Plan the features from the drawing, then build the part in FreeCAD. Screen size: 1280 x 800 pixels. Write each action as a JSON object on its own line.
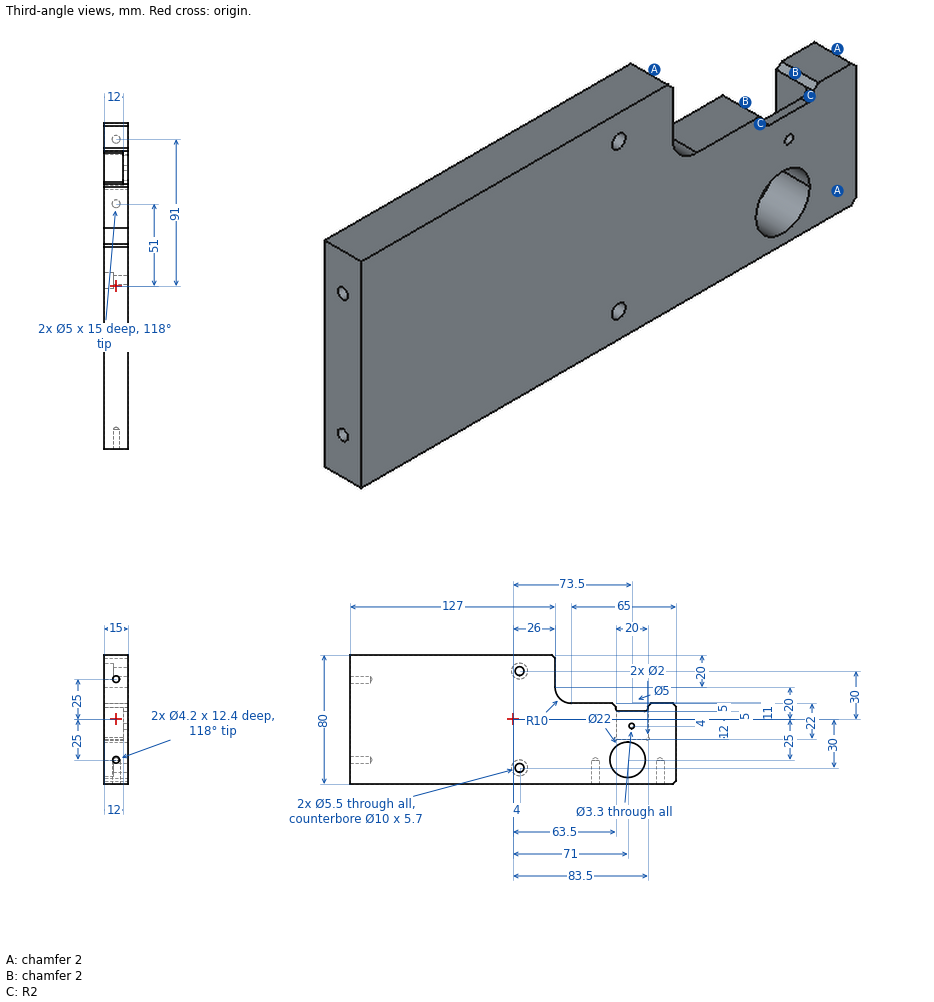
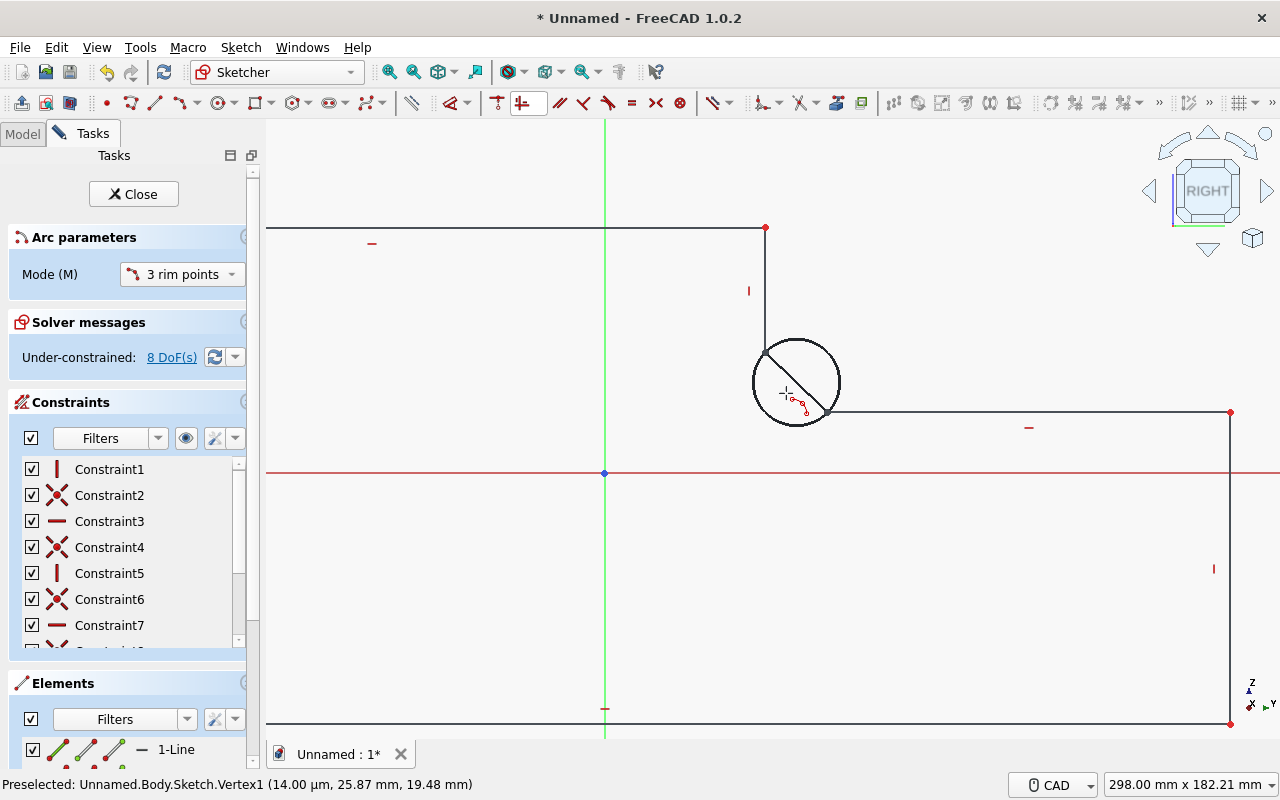
{"action": "left_click", "coordinate": [784, 393]}
{"action": "key", "text": "Escape"}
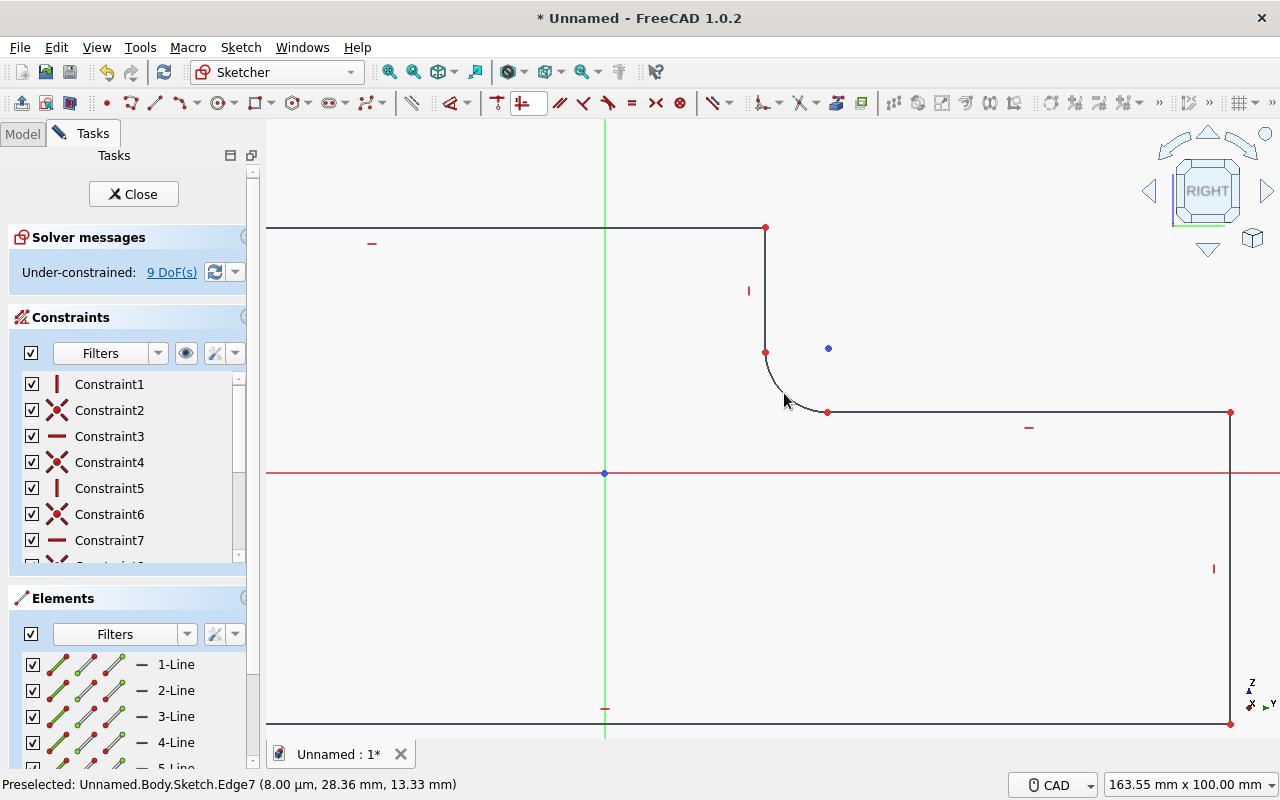
{"action": "left_click", "coordinate": [765, 315]}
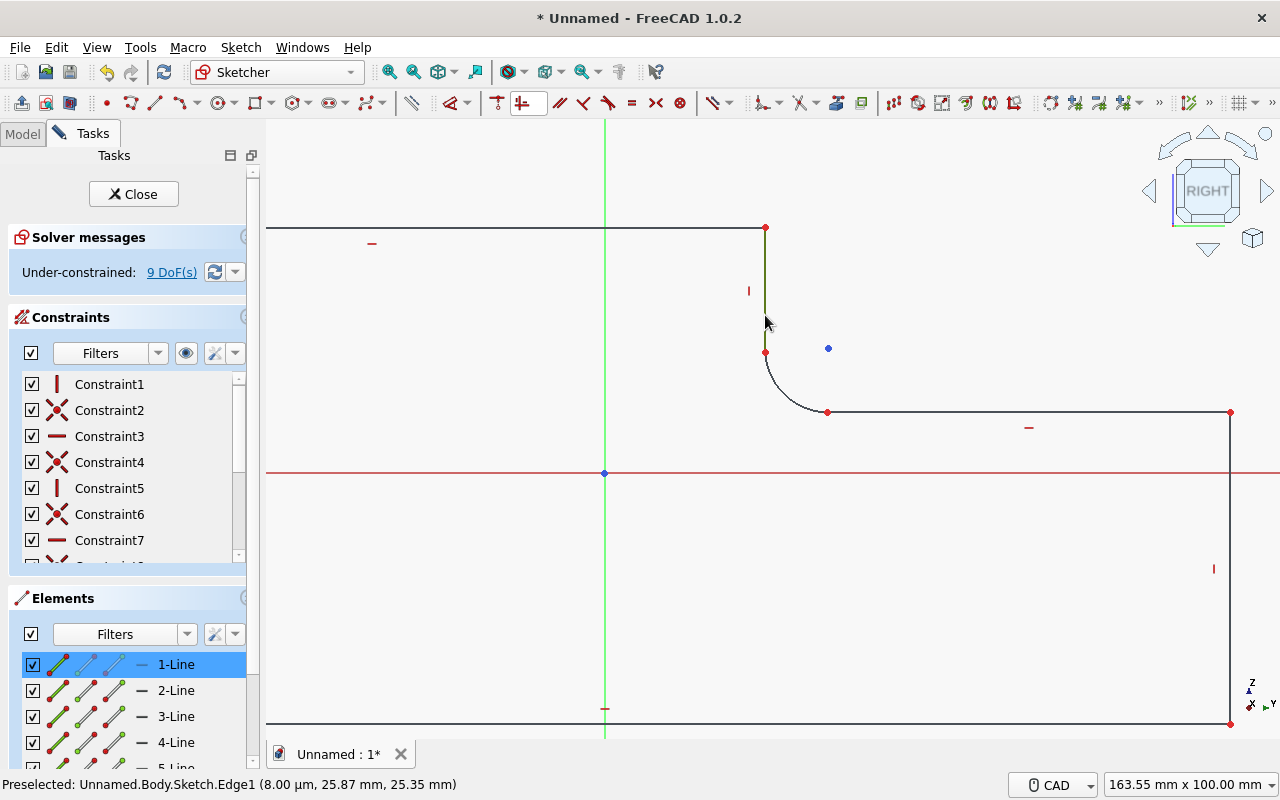
{"action": "left_click", "coordinate": [773, 380]}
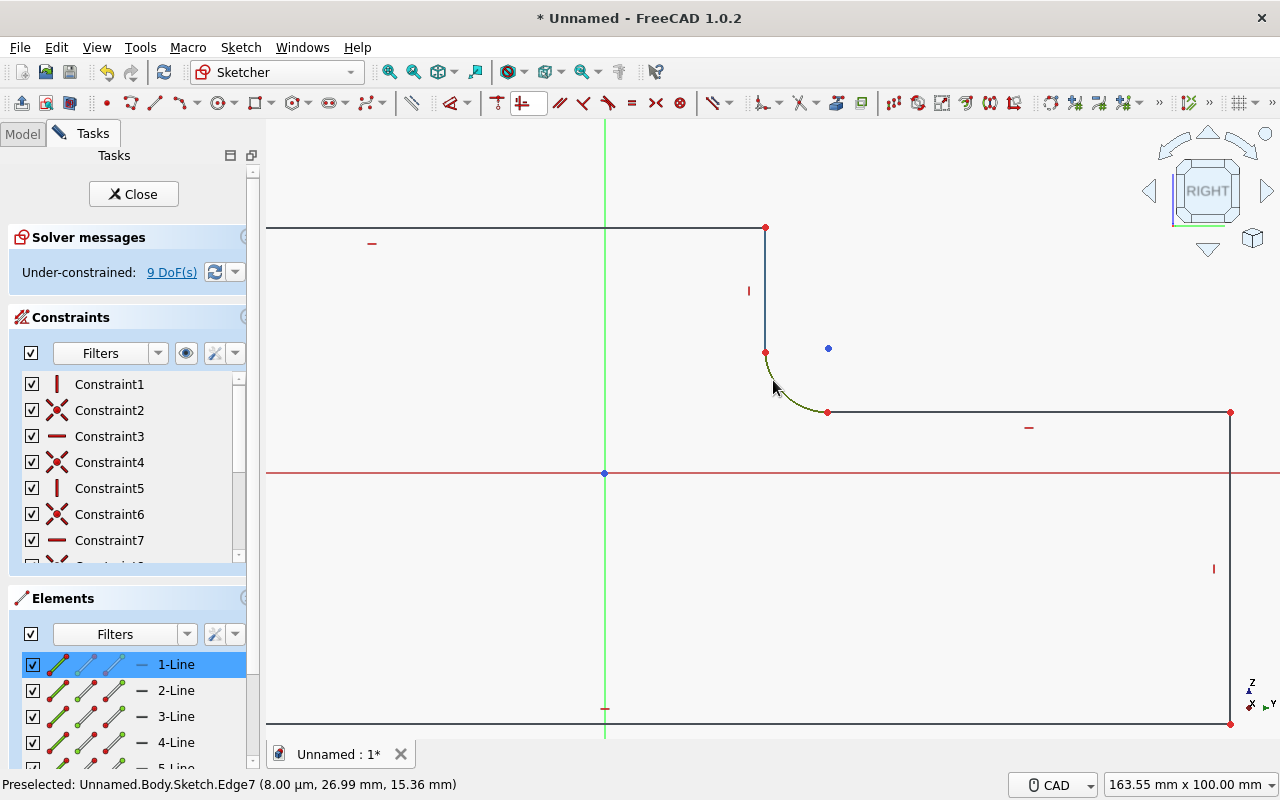
{"action": "left_click", "coordinate": [608, 104]}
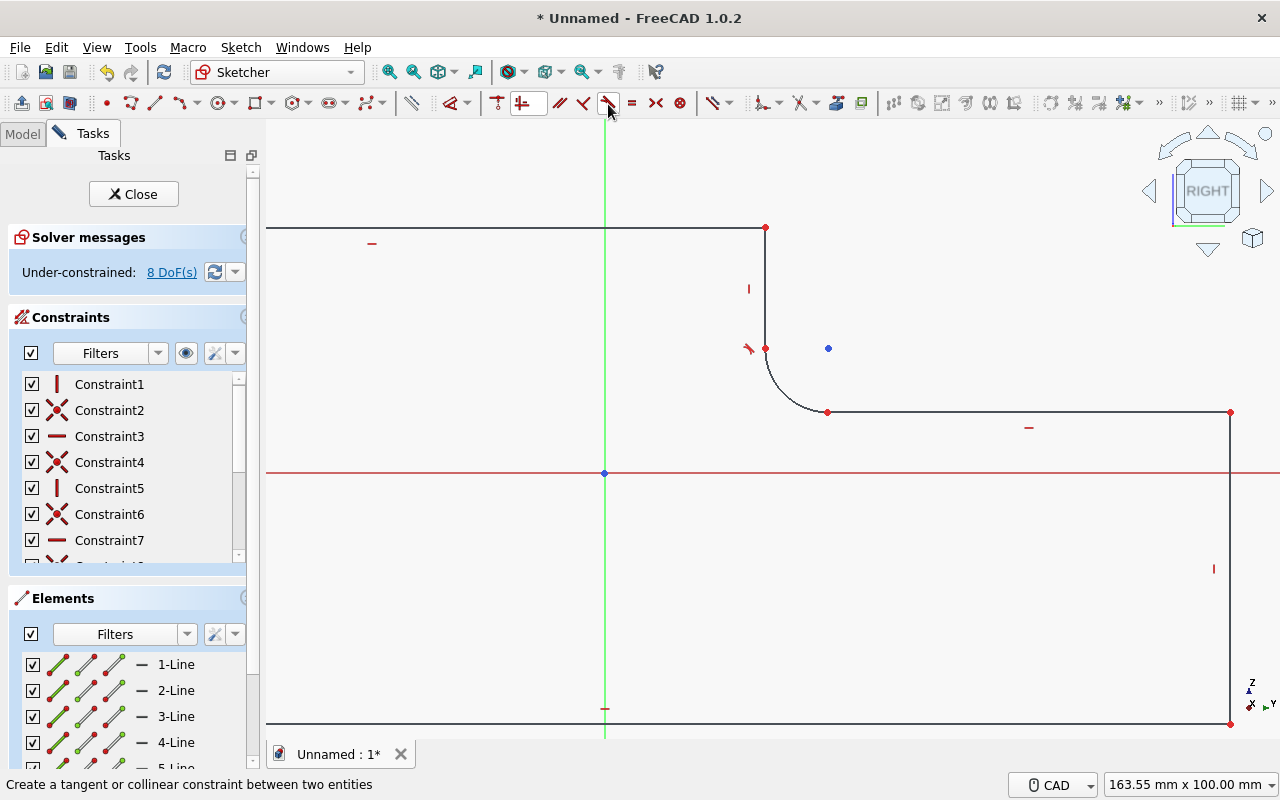
{"action": "left_click", "coordinate": [1110, 412]}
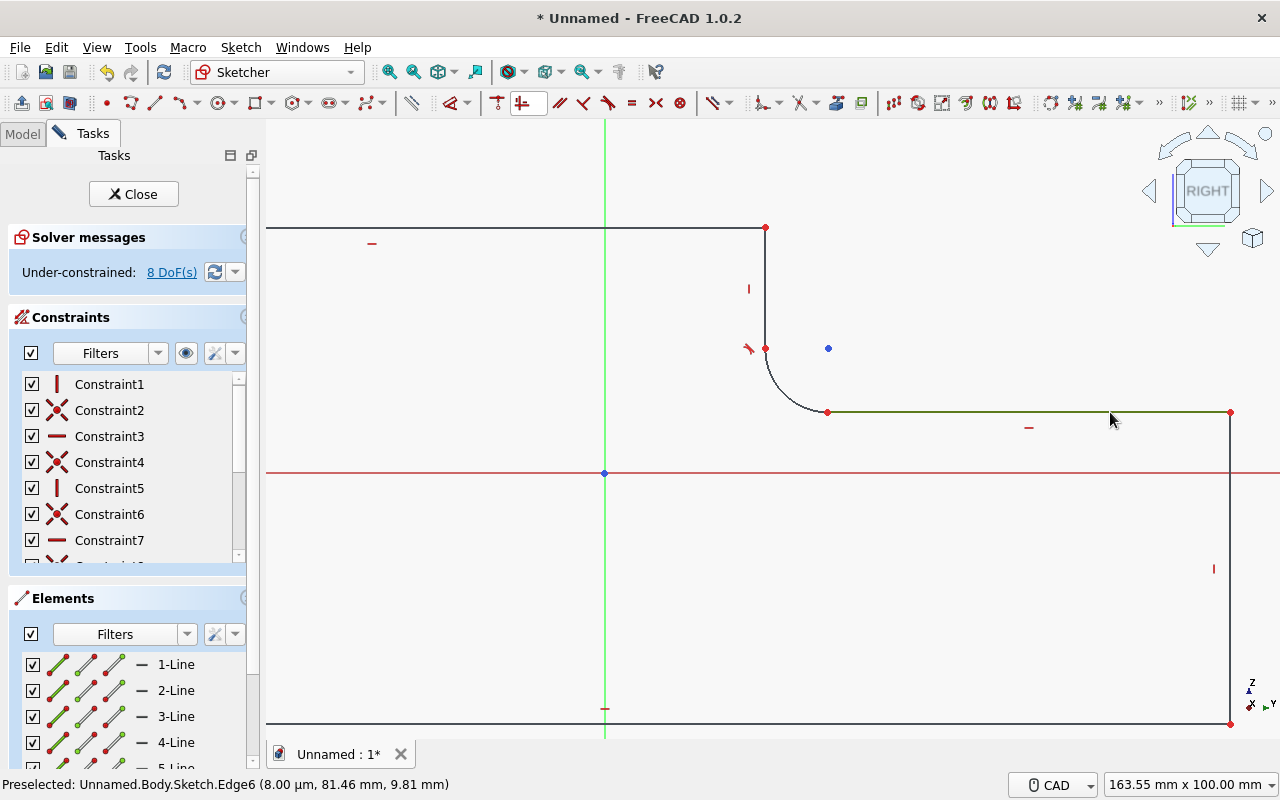
{"action": "left_click", "coordinate": [772, 377]}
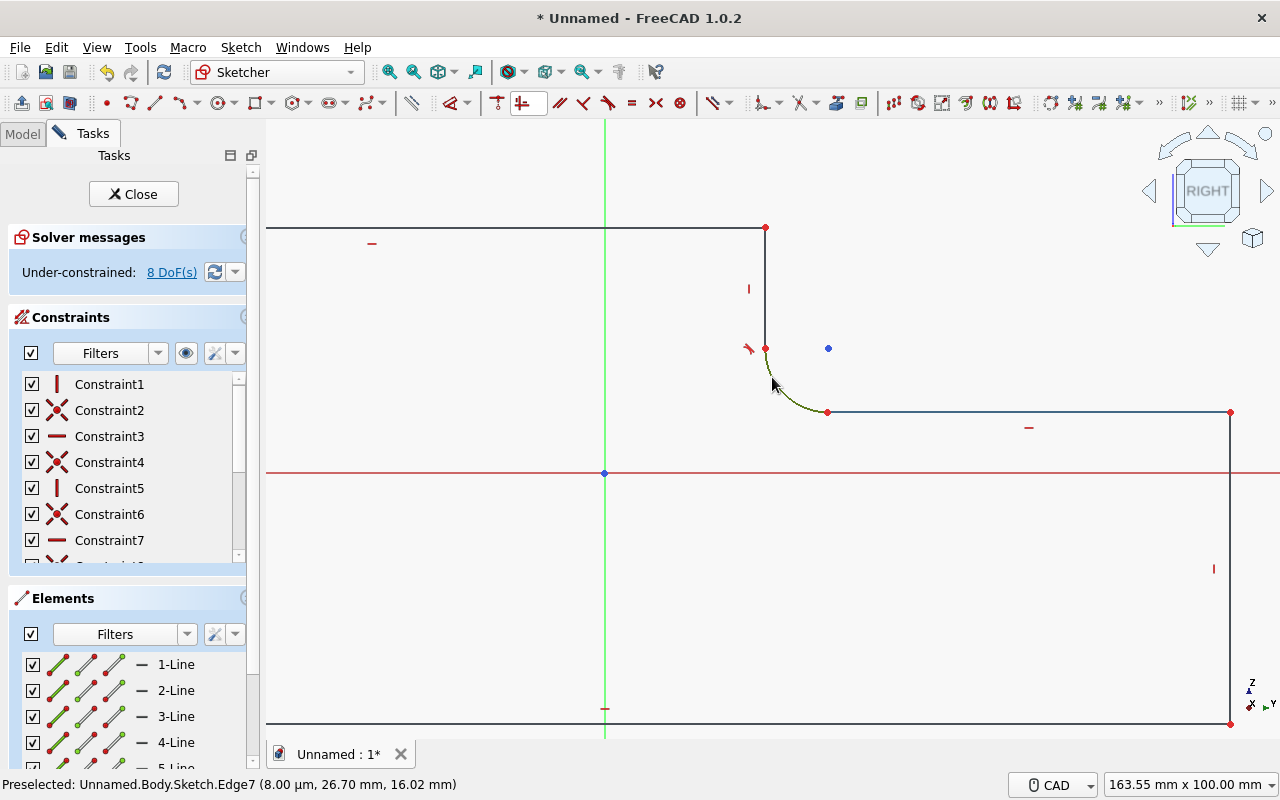
{"action": "left_click", "coordinate": [608, 104]}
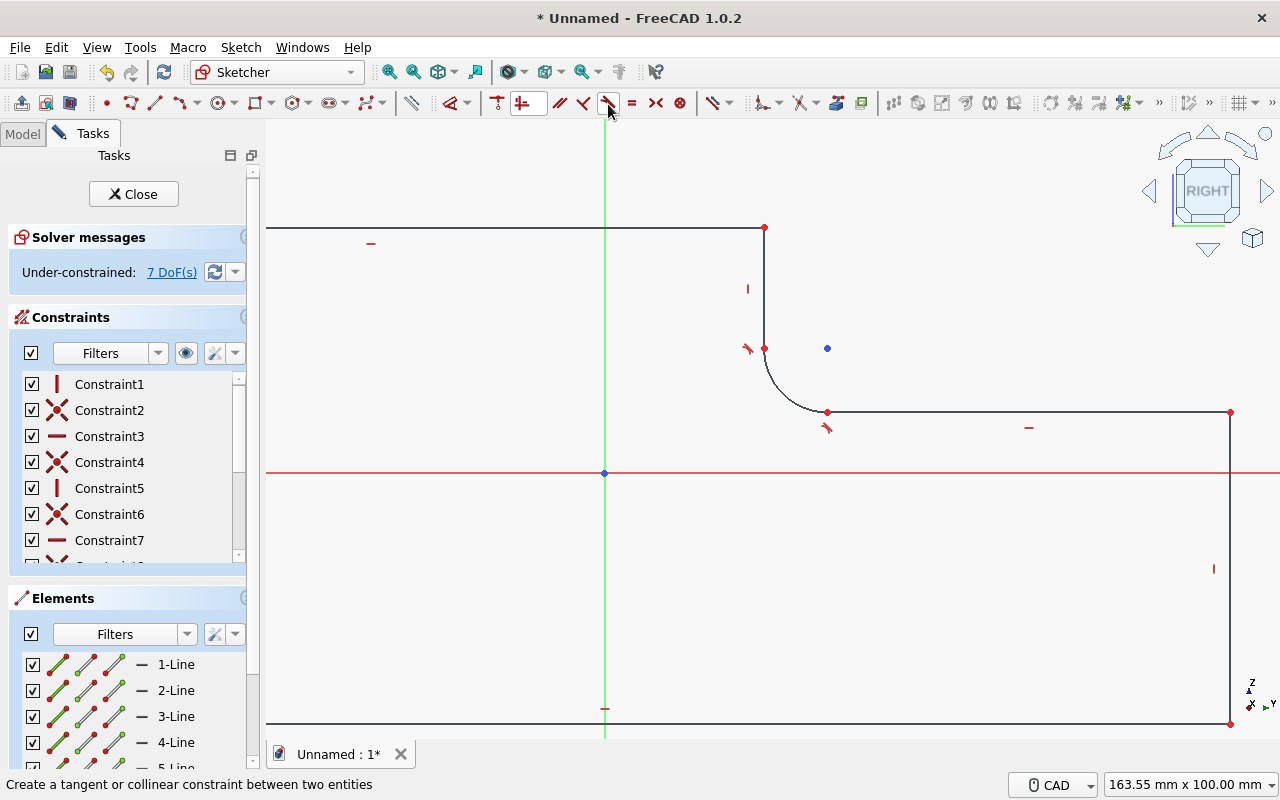
{"action": "left_click", "coordinate": [450, 104]}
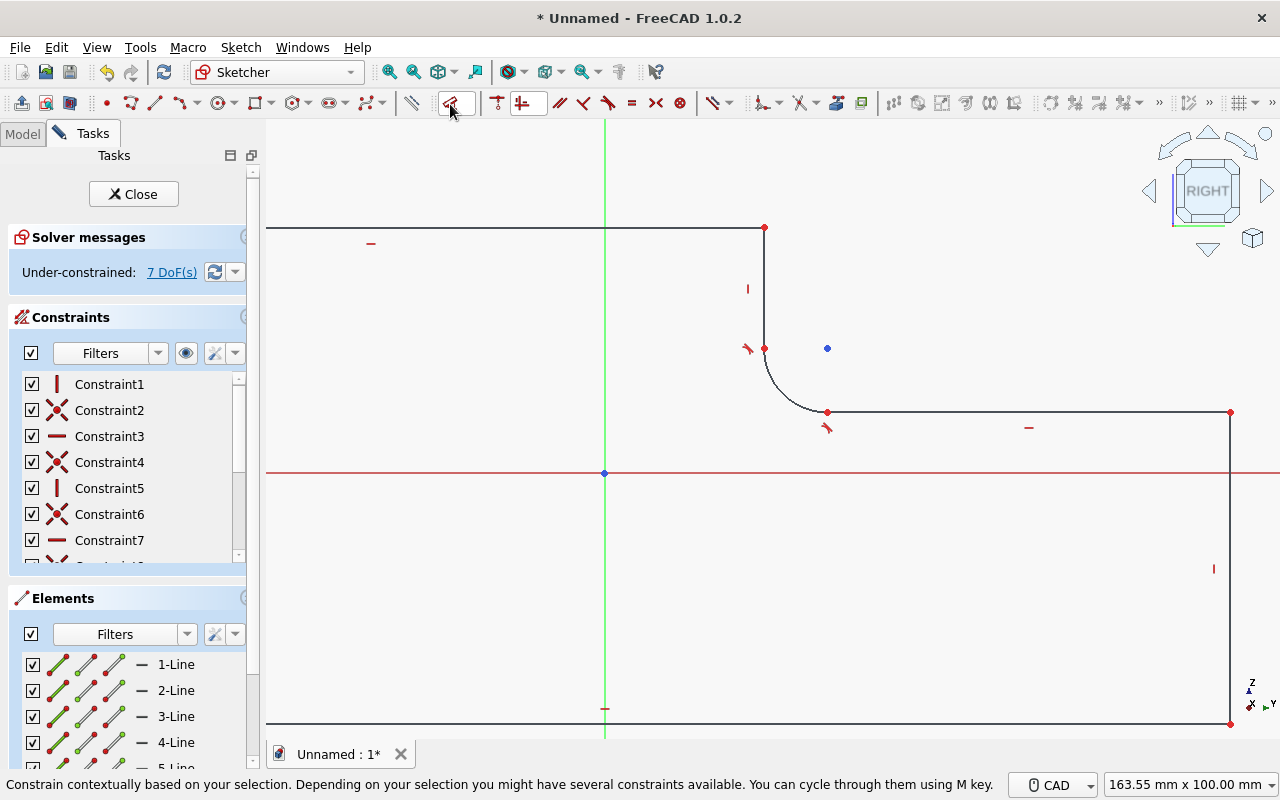
{"action": "left_click", "coordinate": [771, 378]}
{"action": "left_click", "coordinate": [743, 393]}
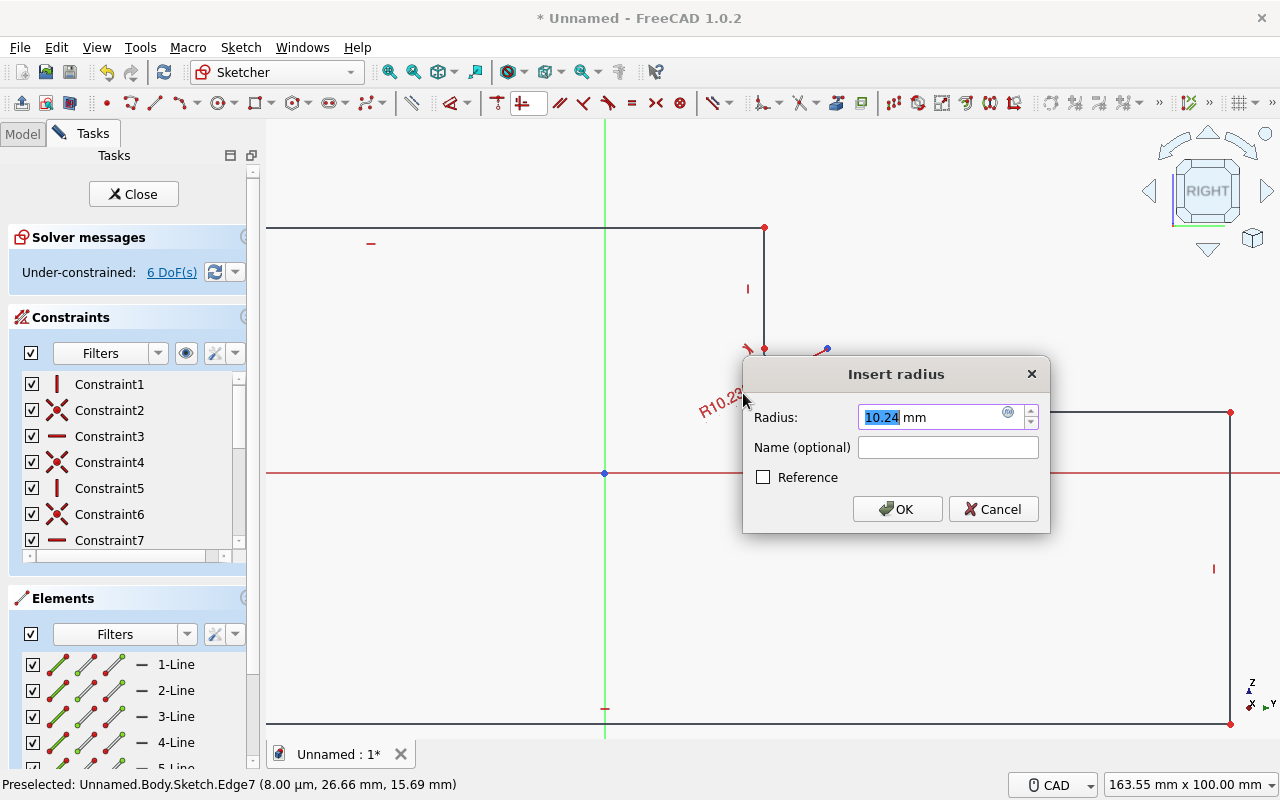
{"action": "type", "text": "10"}
{"action": "key", "text": "Return"}